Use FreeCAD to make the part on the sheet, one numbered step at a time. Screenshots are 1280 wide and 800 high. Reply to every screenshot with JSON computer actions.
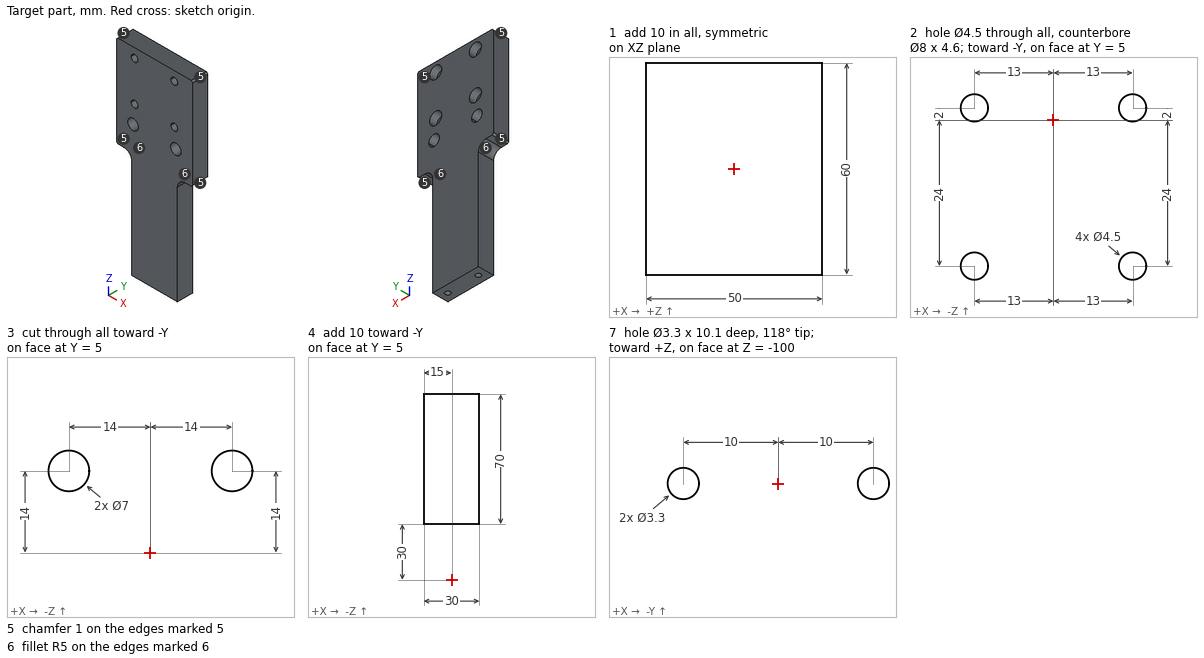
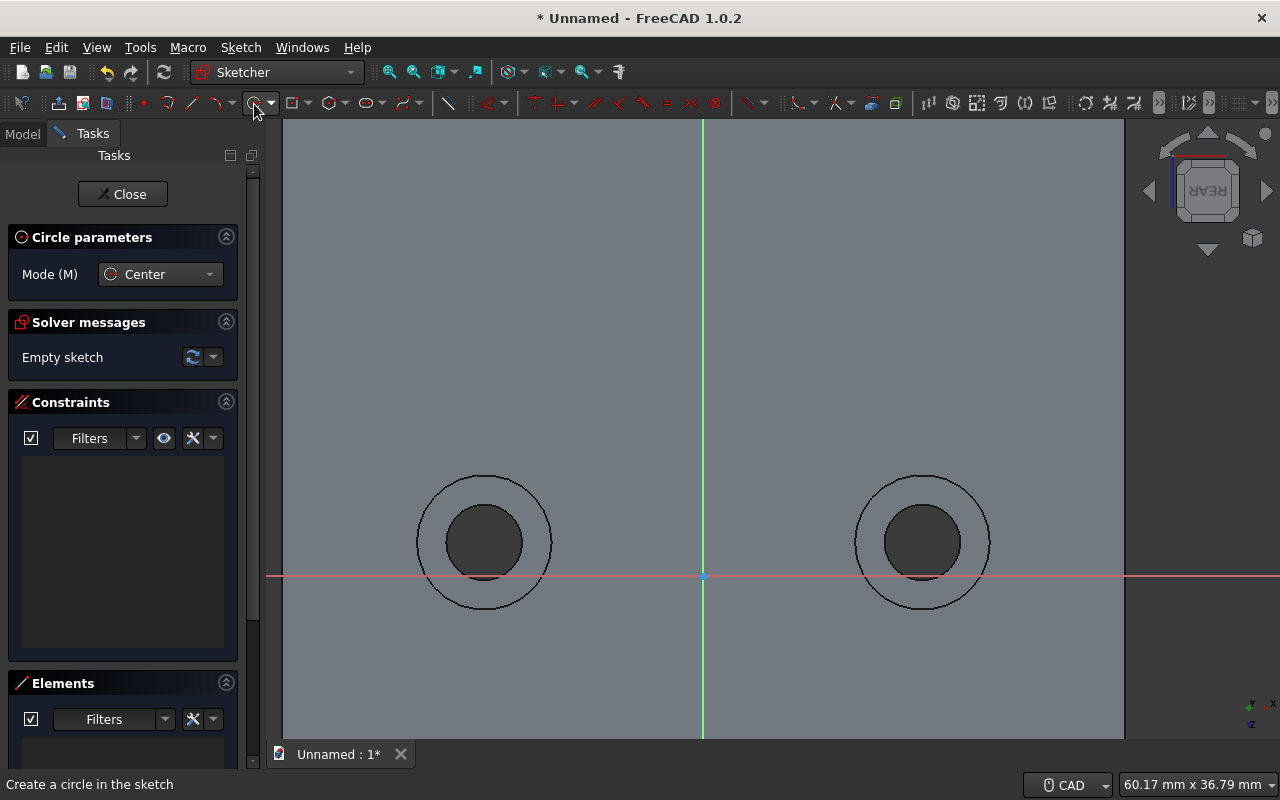
{"action": "left_click", "coordinate": [467, 340]}
{"action": "mouse_move", "coordinate": [509, 298]}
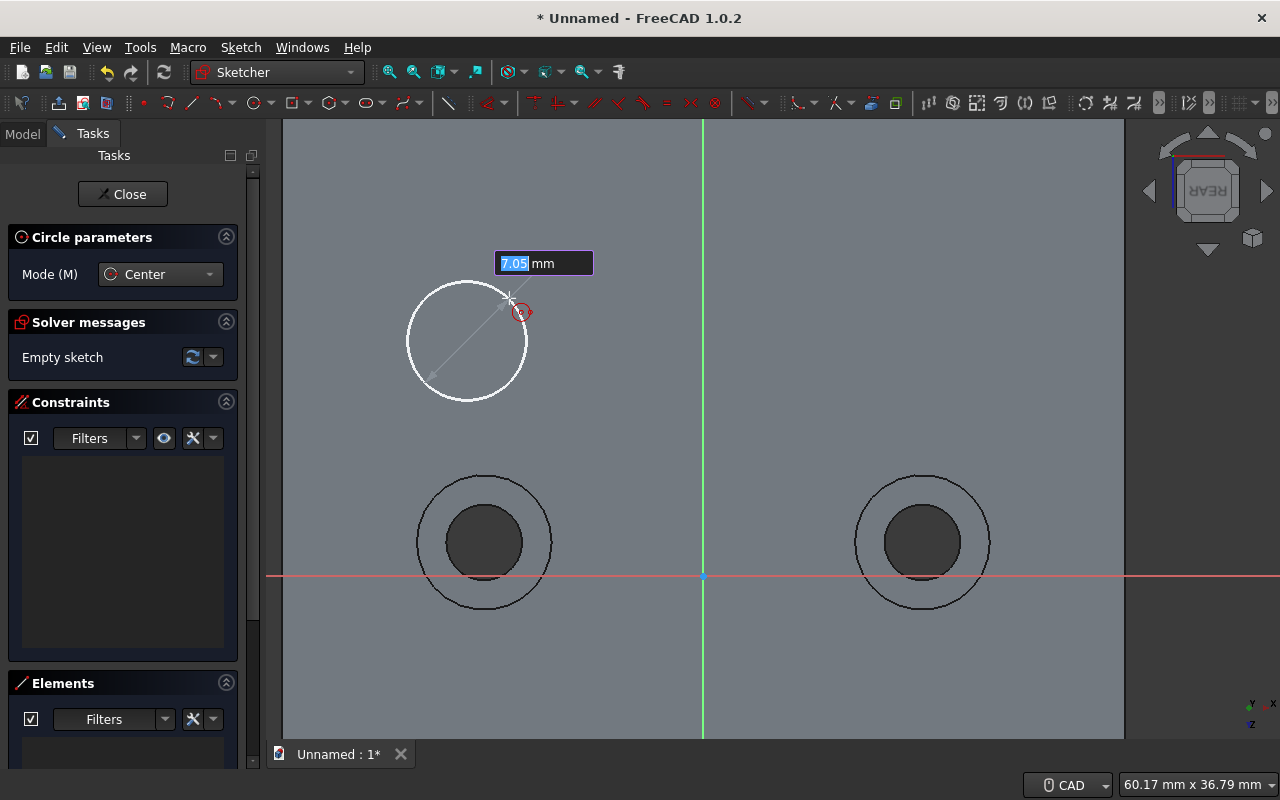
{"action": "type", "text": "7"}
{"action": "key", "text": "Return"}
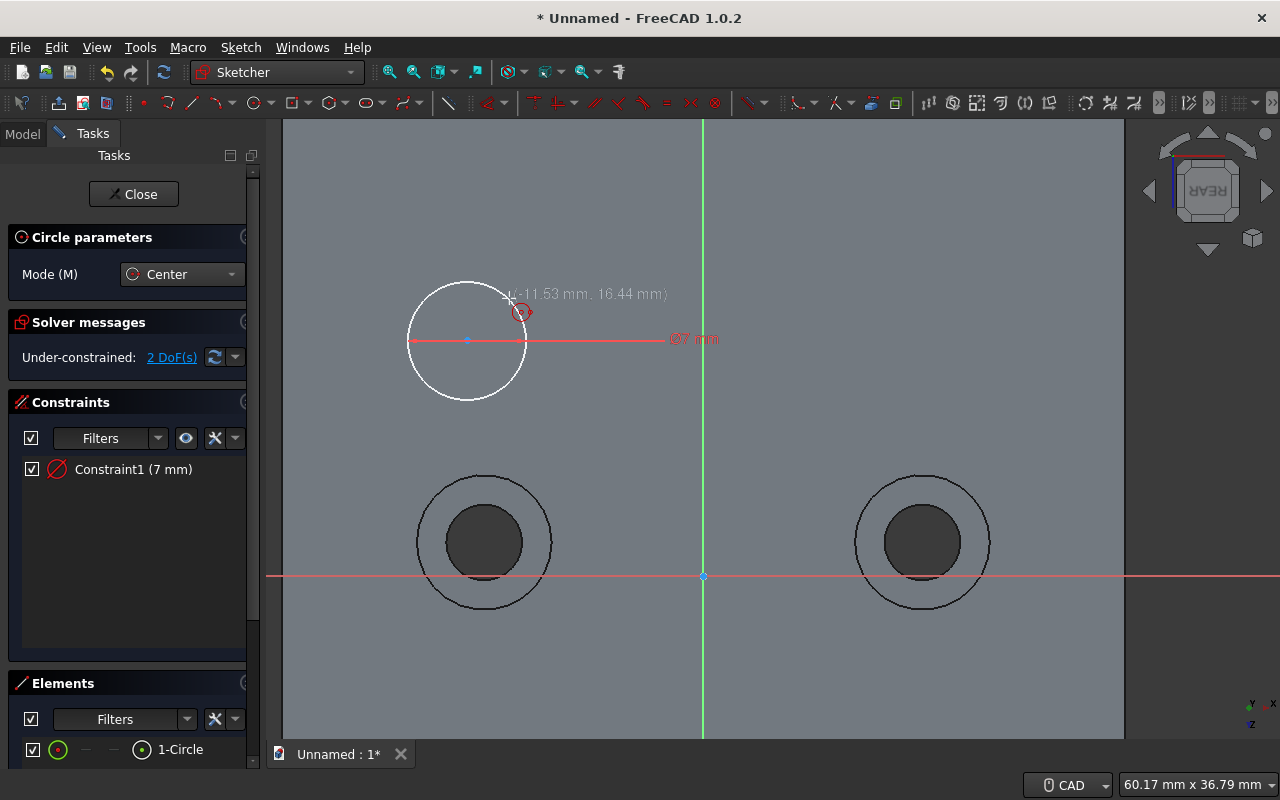
{"action": "left_click", "coordinate": [939, 340]}
{"action": "mouse_move", "coordinate": [981, 298]}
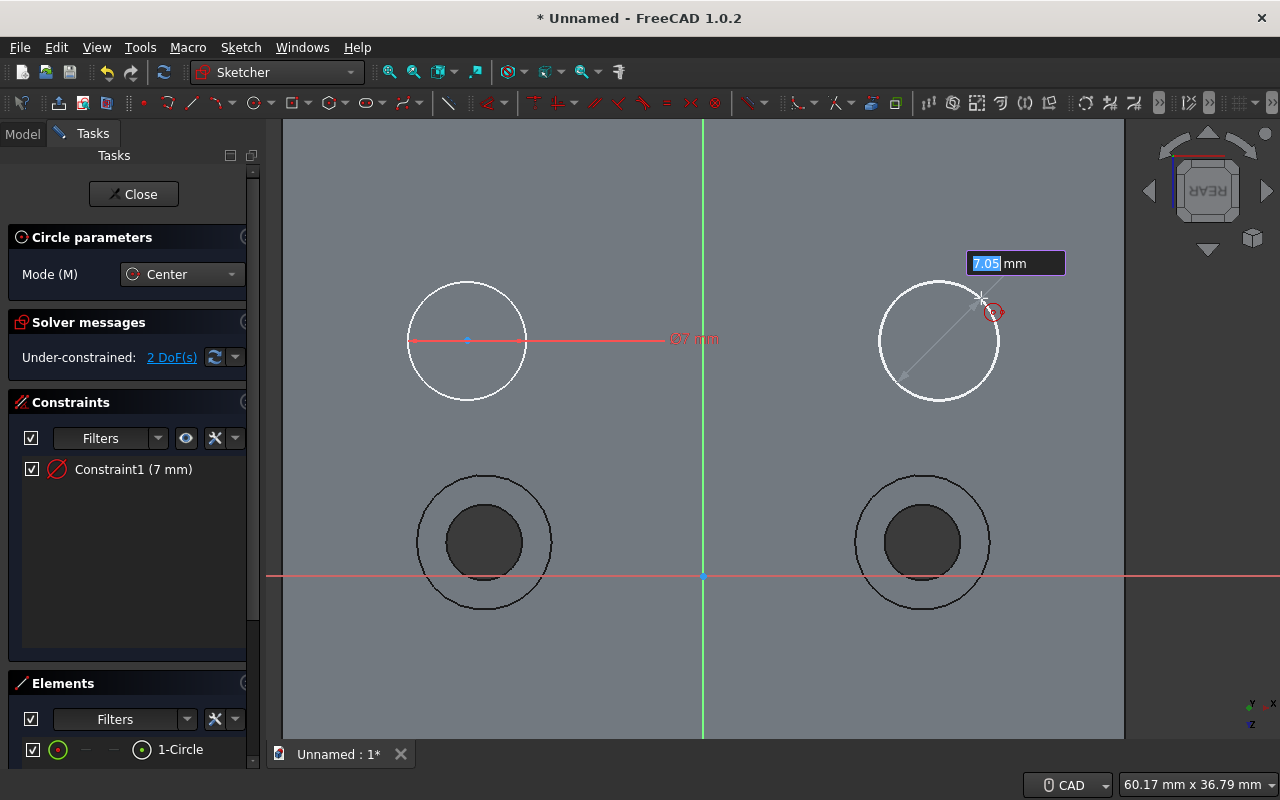
{"action": "type", "text": "7"}
{"action": "key", "text": "Return"}
{"action": "key", "text": "Escape"}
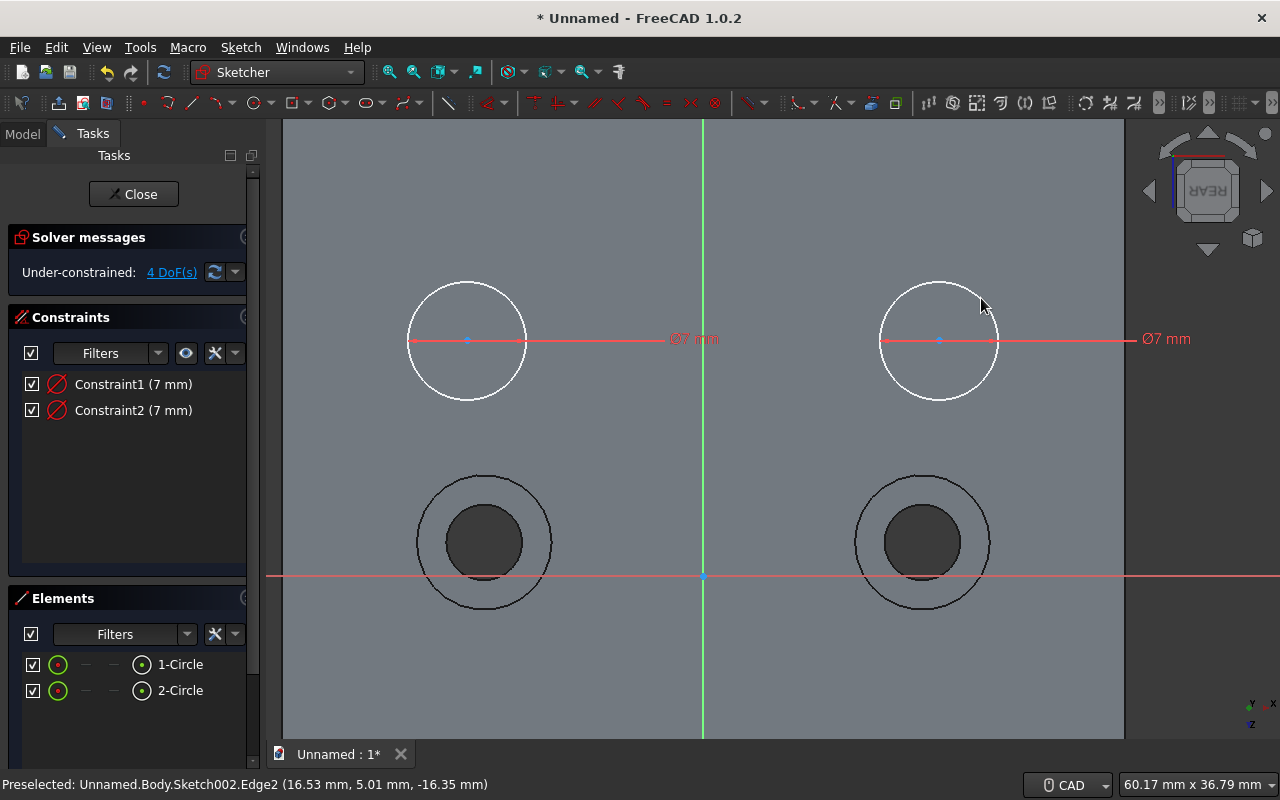
{"action": "left_click", "coordinate": [488, 104]}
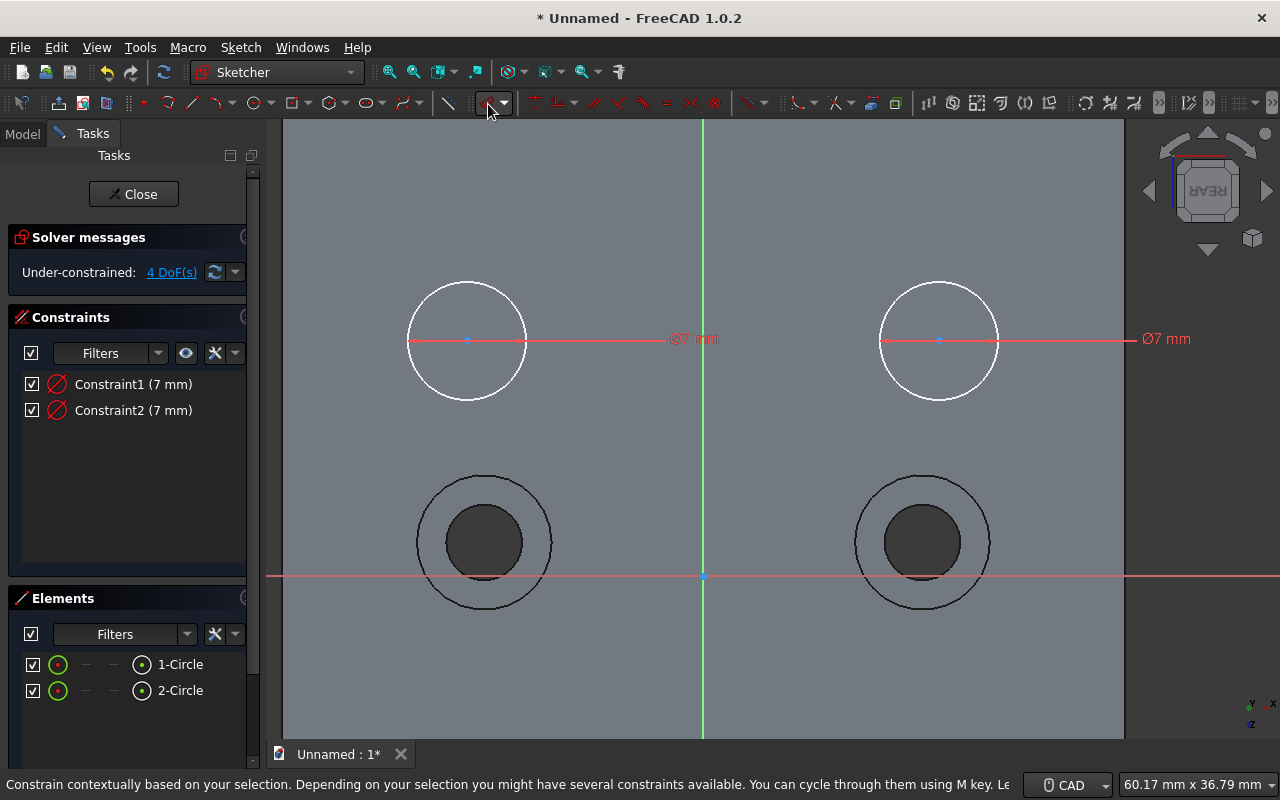
{"action": "left_click", "coordinate": [467, 341]}
{"action": "left_click", "coordinate": [585, 610]}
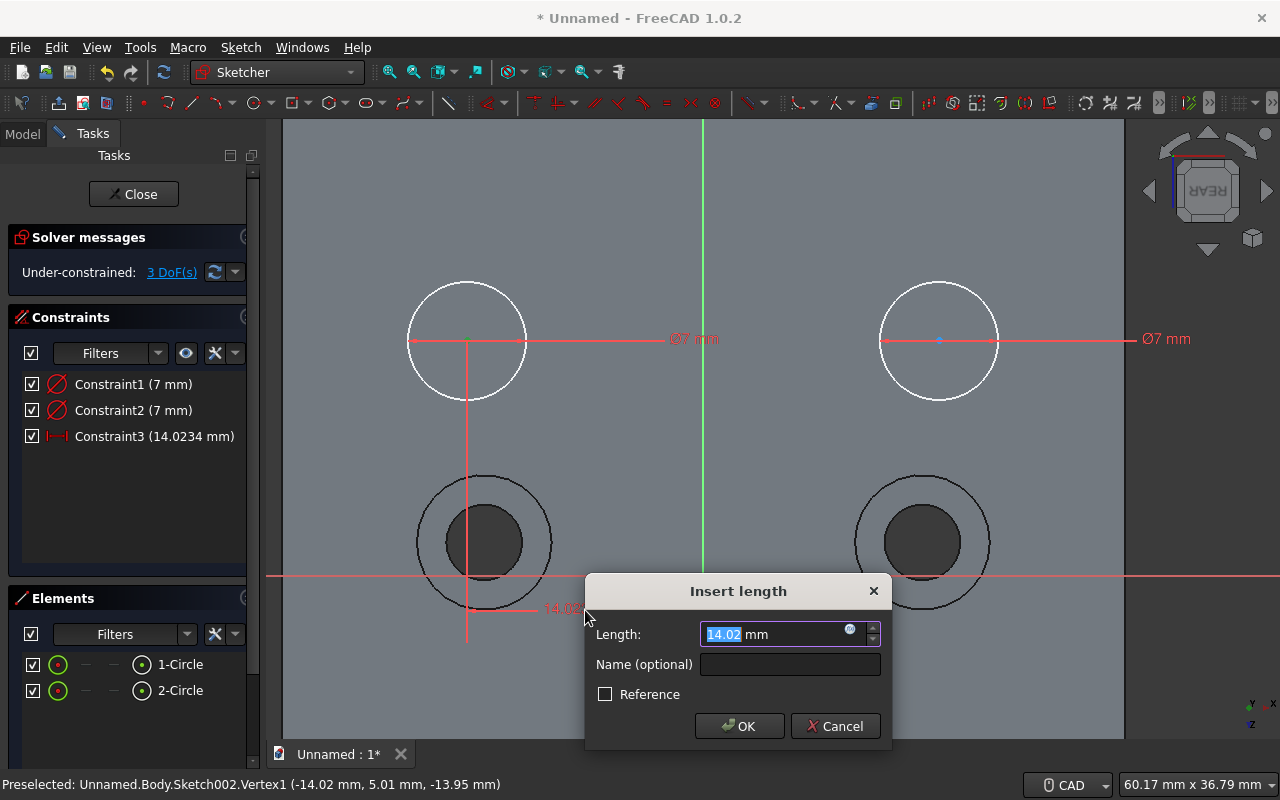
{"action": "type", "text": "14"}
{"action": "key", "text": "Return"}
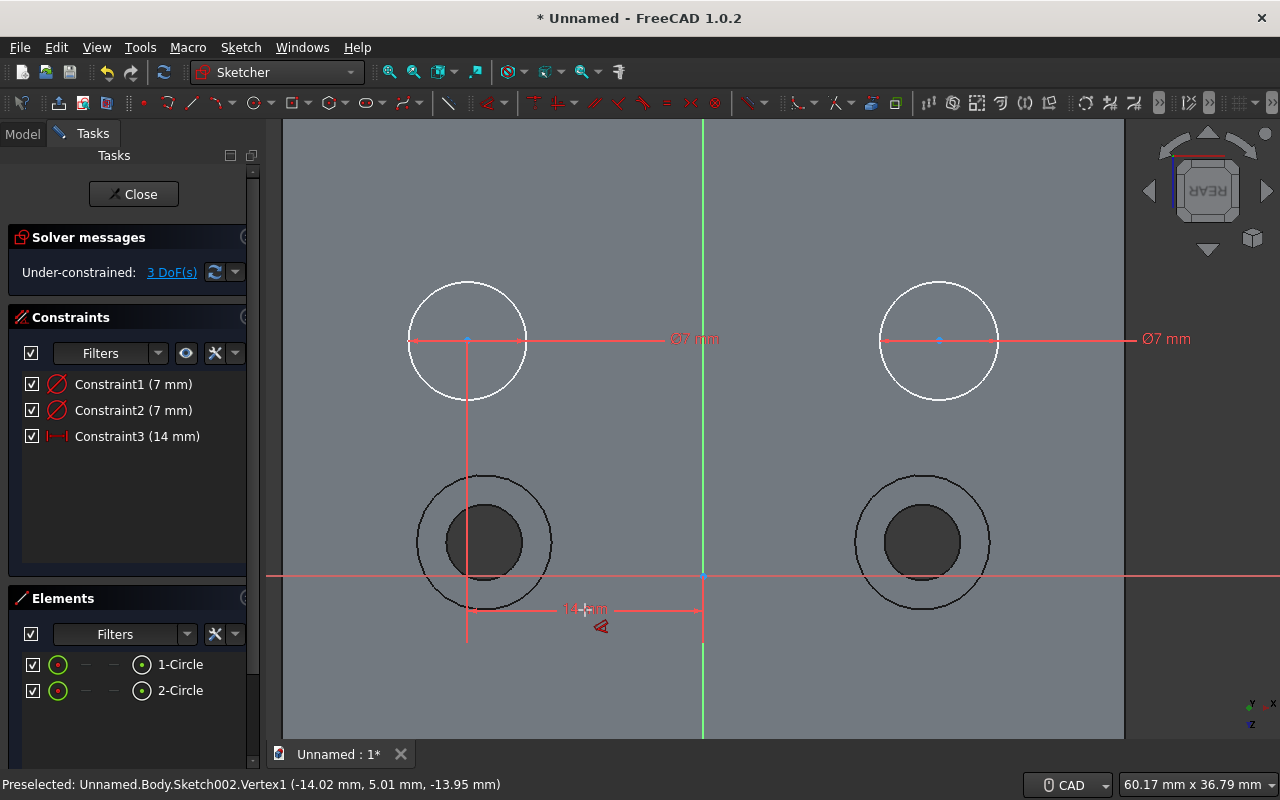
{"action": "left_click", "coordinate": [467, 341]}
{"action": "left_click", "coordinate": [433, 459]}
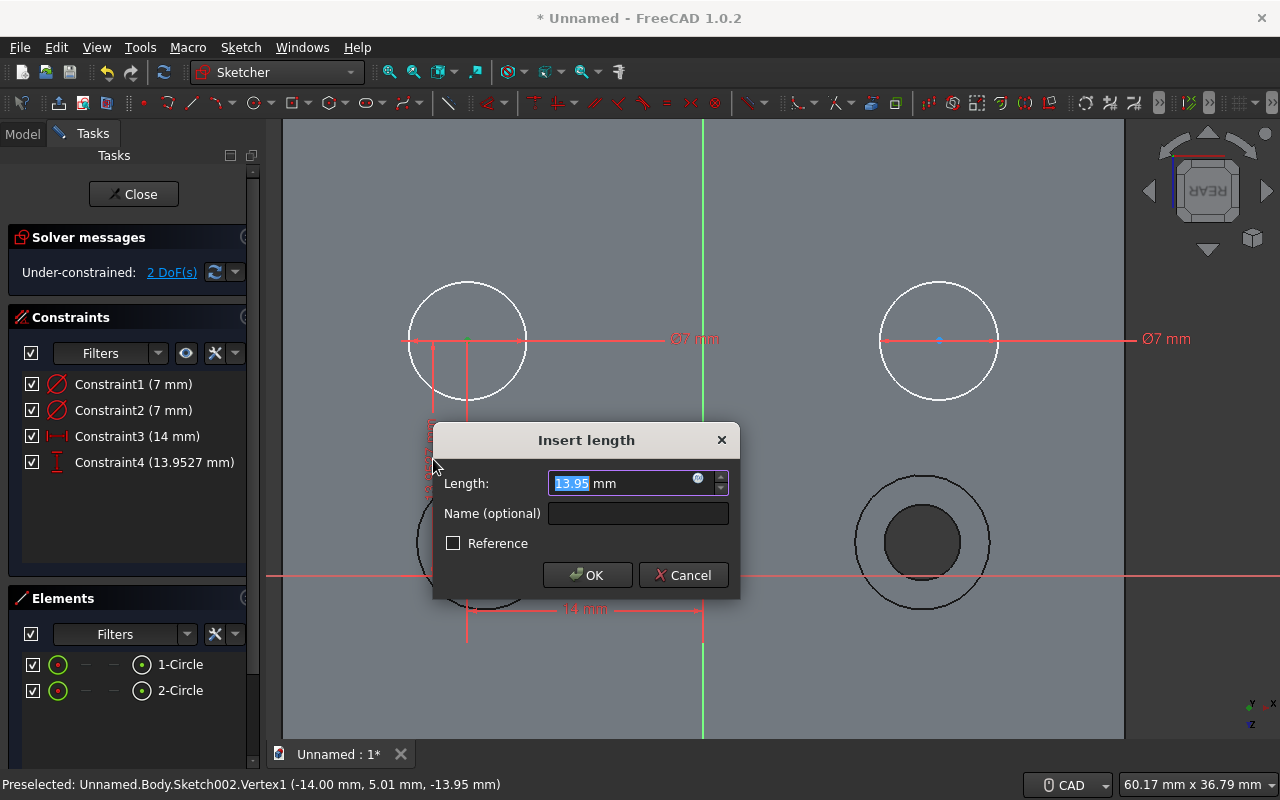
{"action": "type", "text": "14"}
{"action": "key", "text": "Return"}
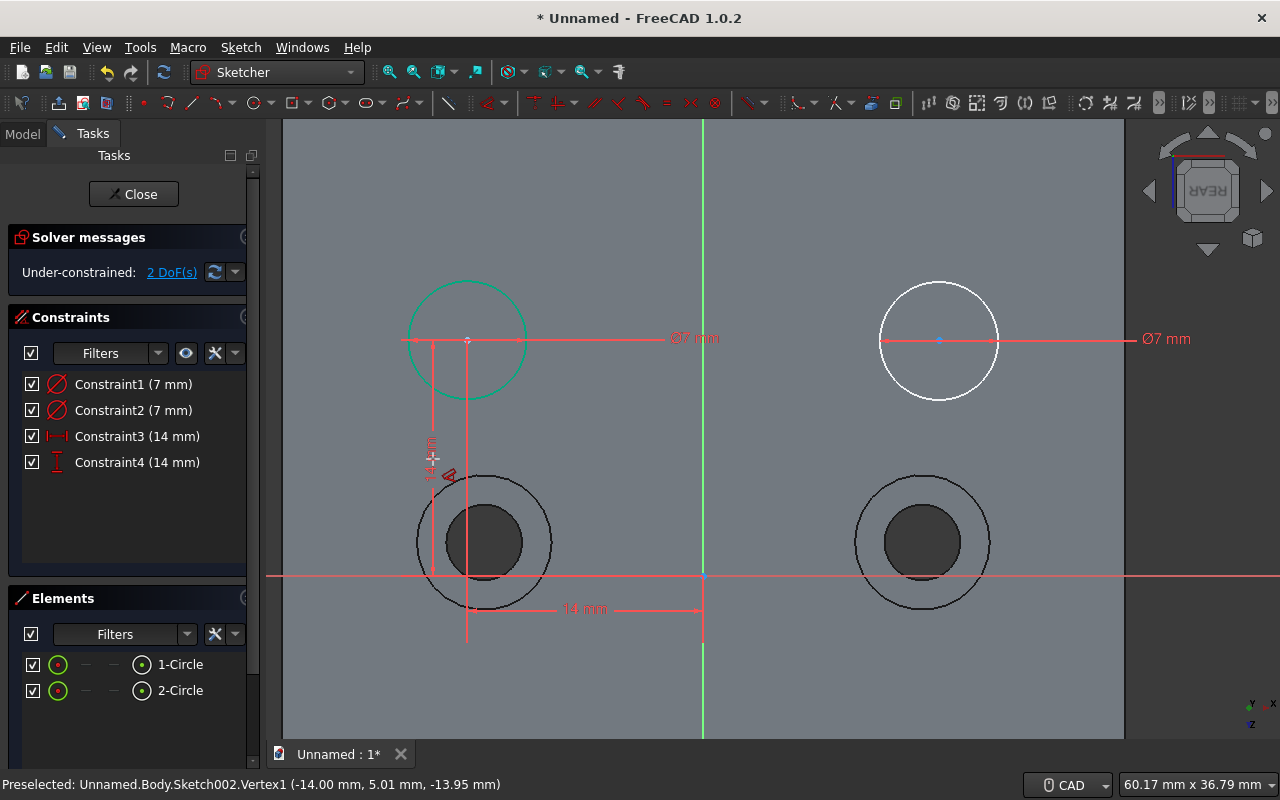
{"action": "left_click", "coordinate": [939, 341]}
{"action": "left_click", "coordinate": [821, 610]}